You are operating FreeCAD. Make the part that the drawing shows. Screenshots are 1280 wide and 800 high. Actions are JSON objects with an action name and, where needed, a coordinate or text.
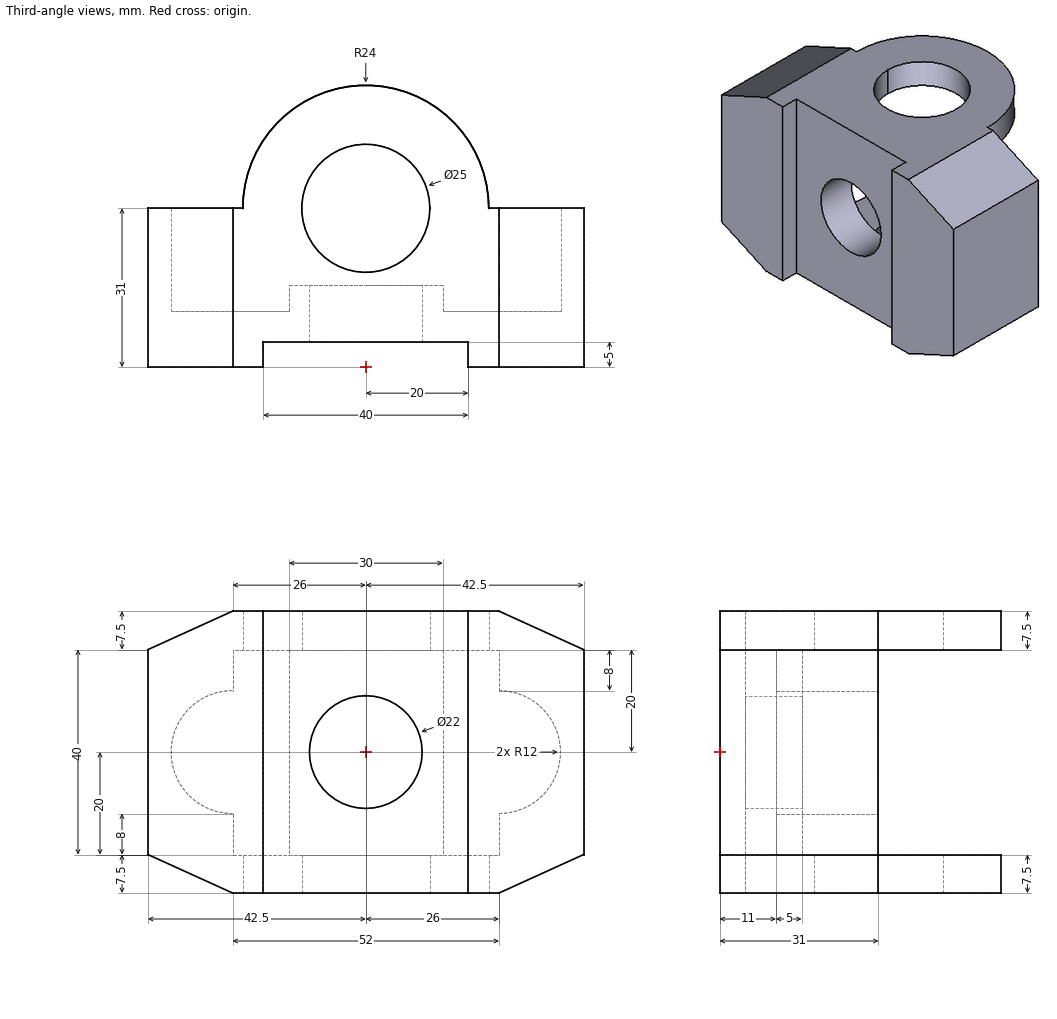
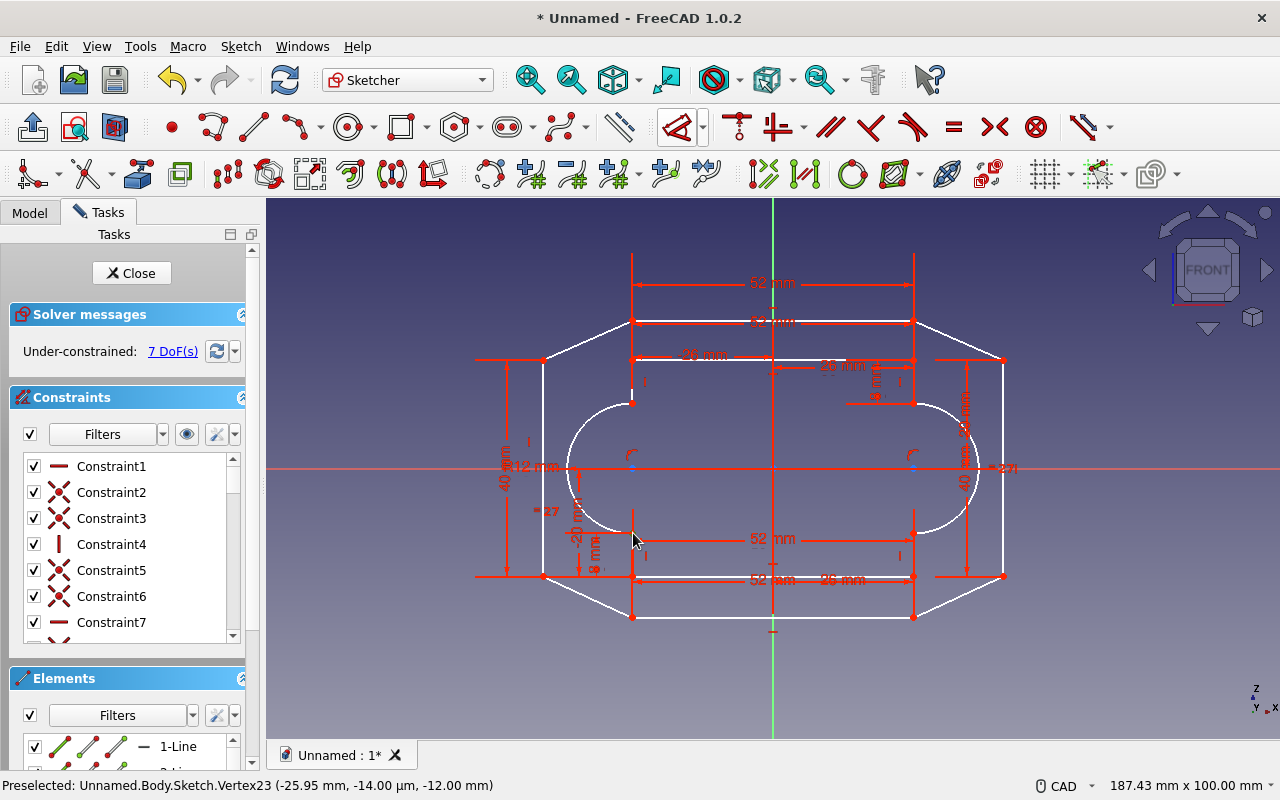
{"action": "key", "text": "l"}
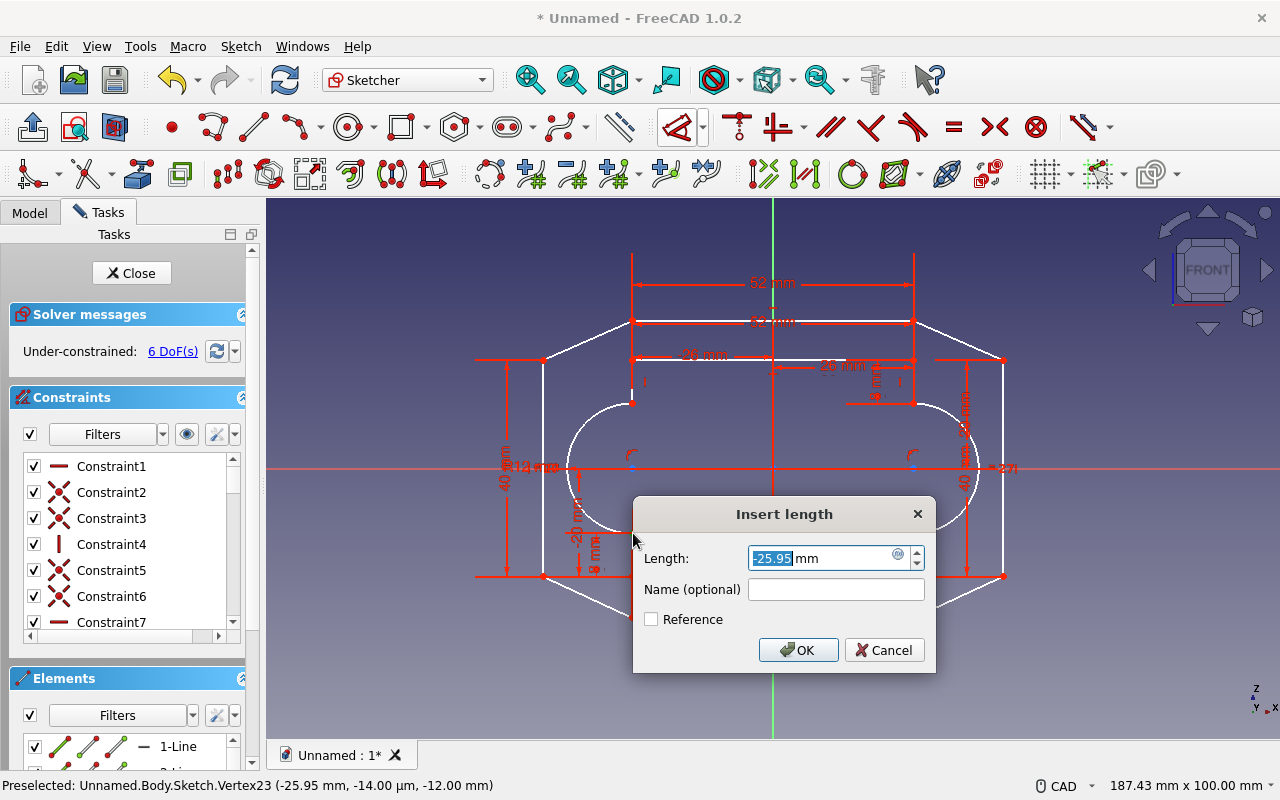
{"action": "type", "text": "-26"}
{"action": "key", "text": "Return"}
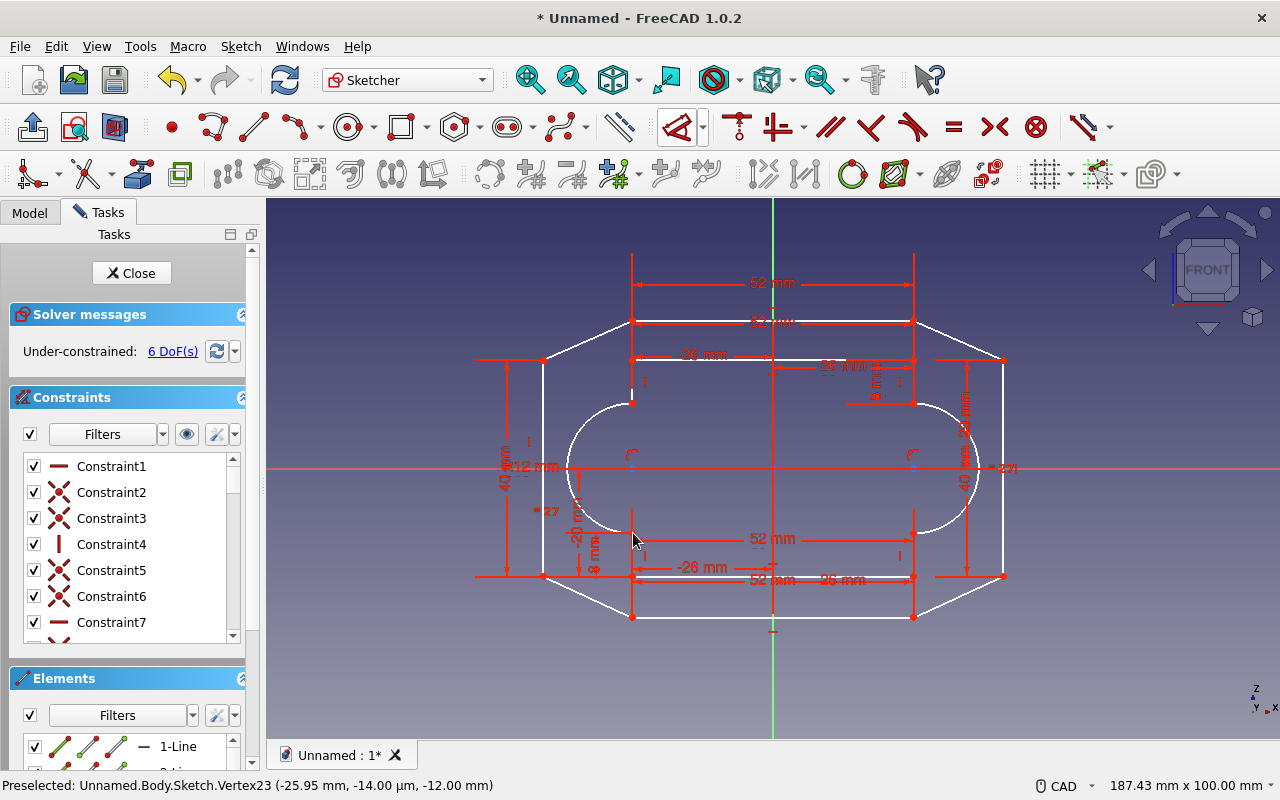
{"action": "left_click", "coordinate": [632, 468]}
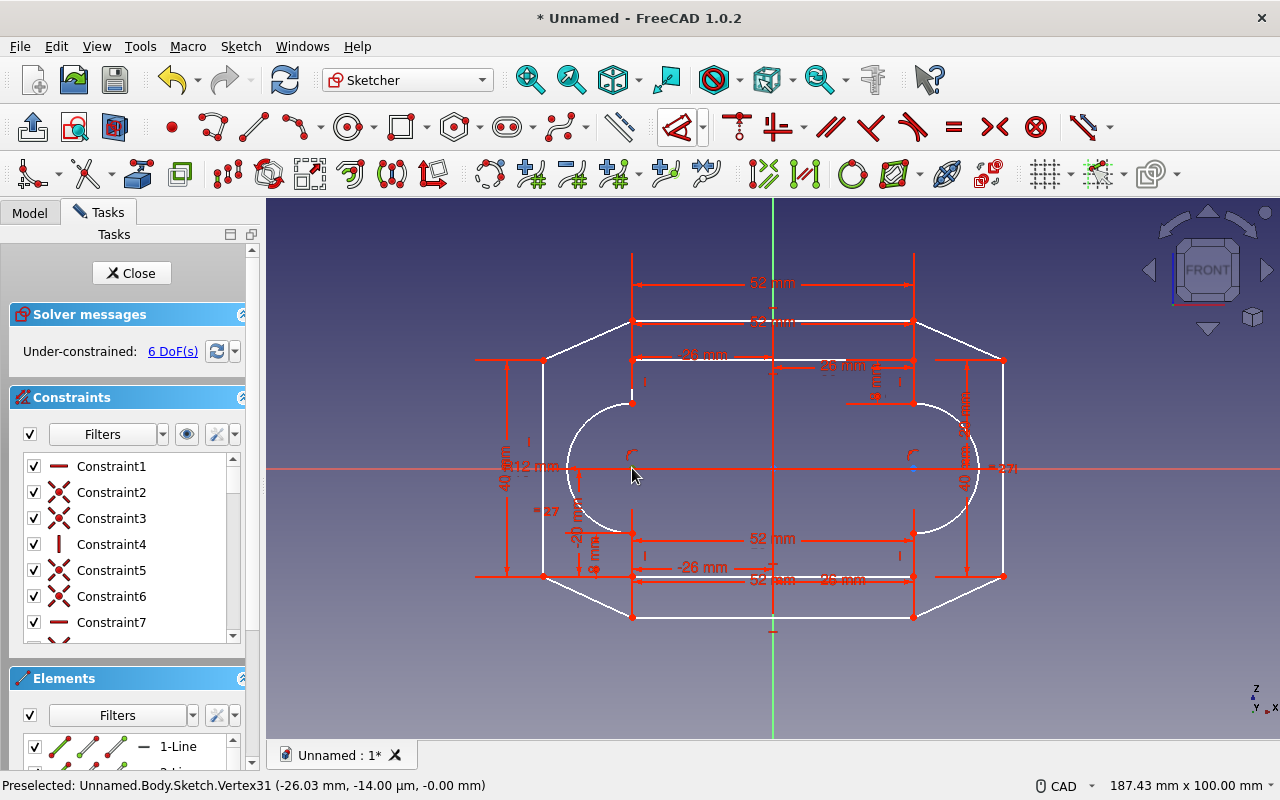
{"action": "left_click", "coordinate": [702, 128]}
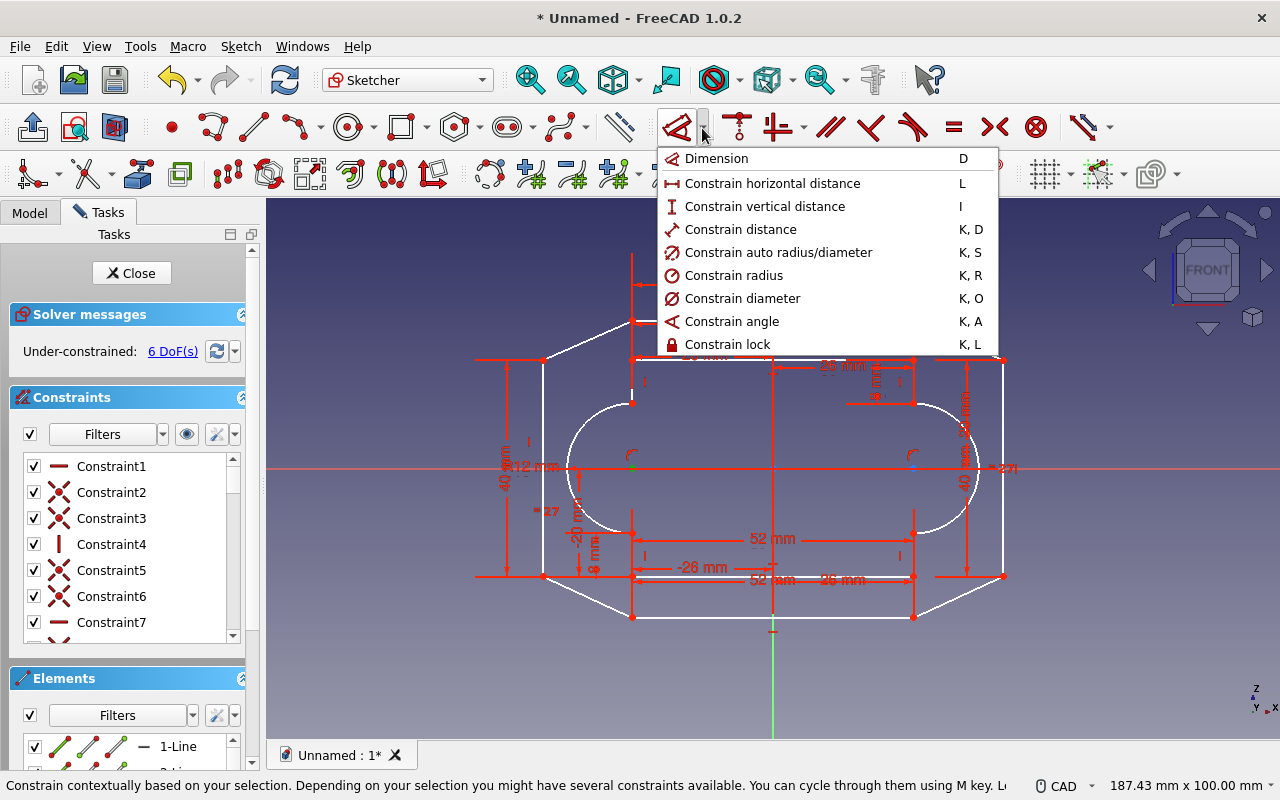
{"action": "left_click", "coordinate": [828, 184]}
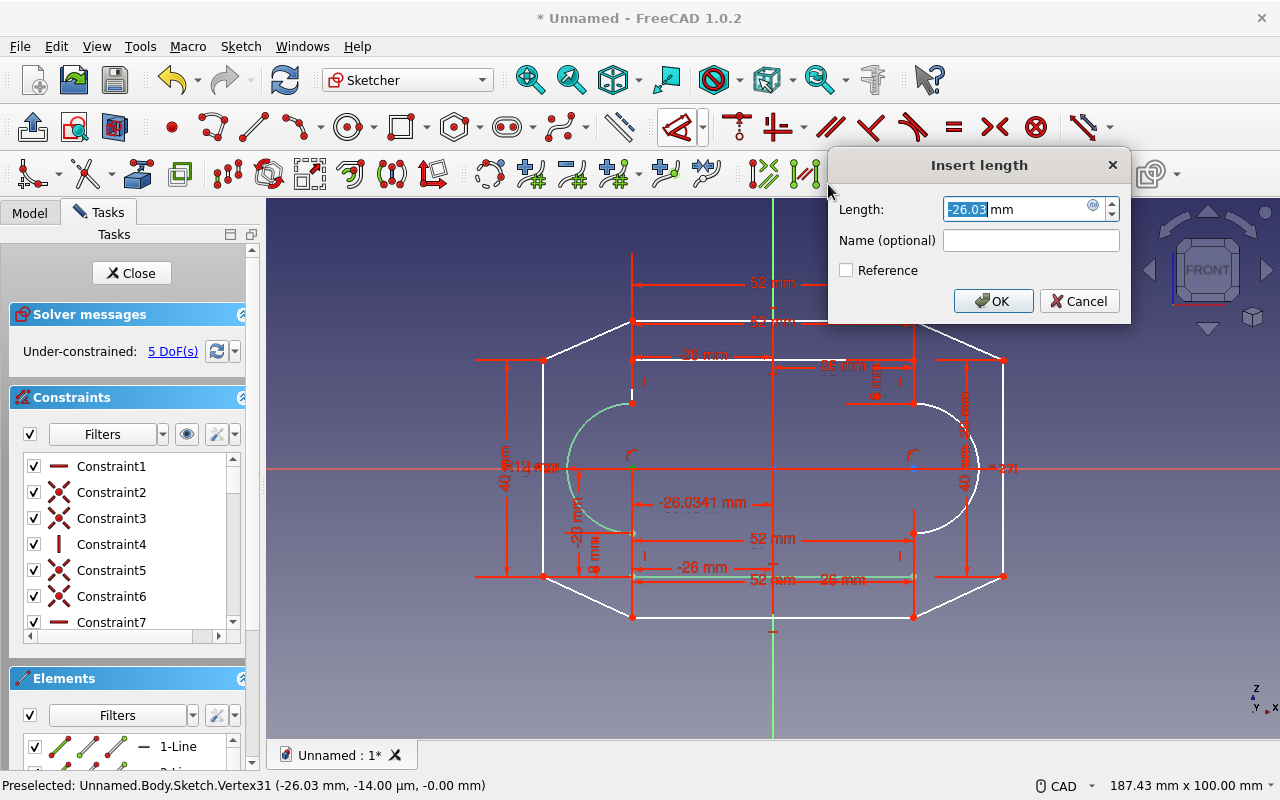
{"action": "type", "text": "-26"}
{"action": "key", "text": "Return"}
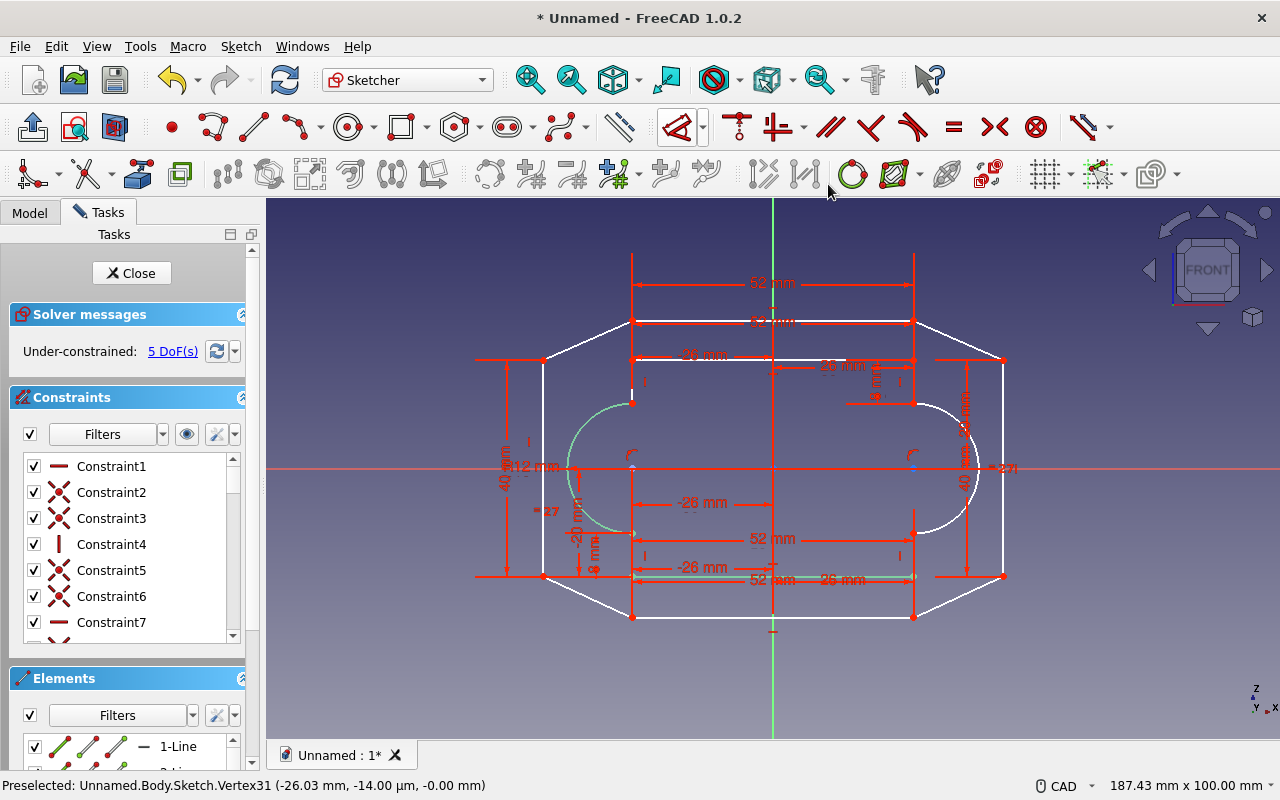
{"action": "left_click", "coordinate": [914, 468]}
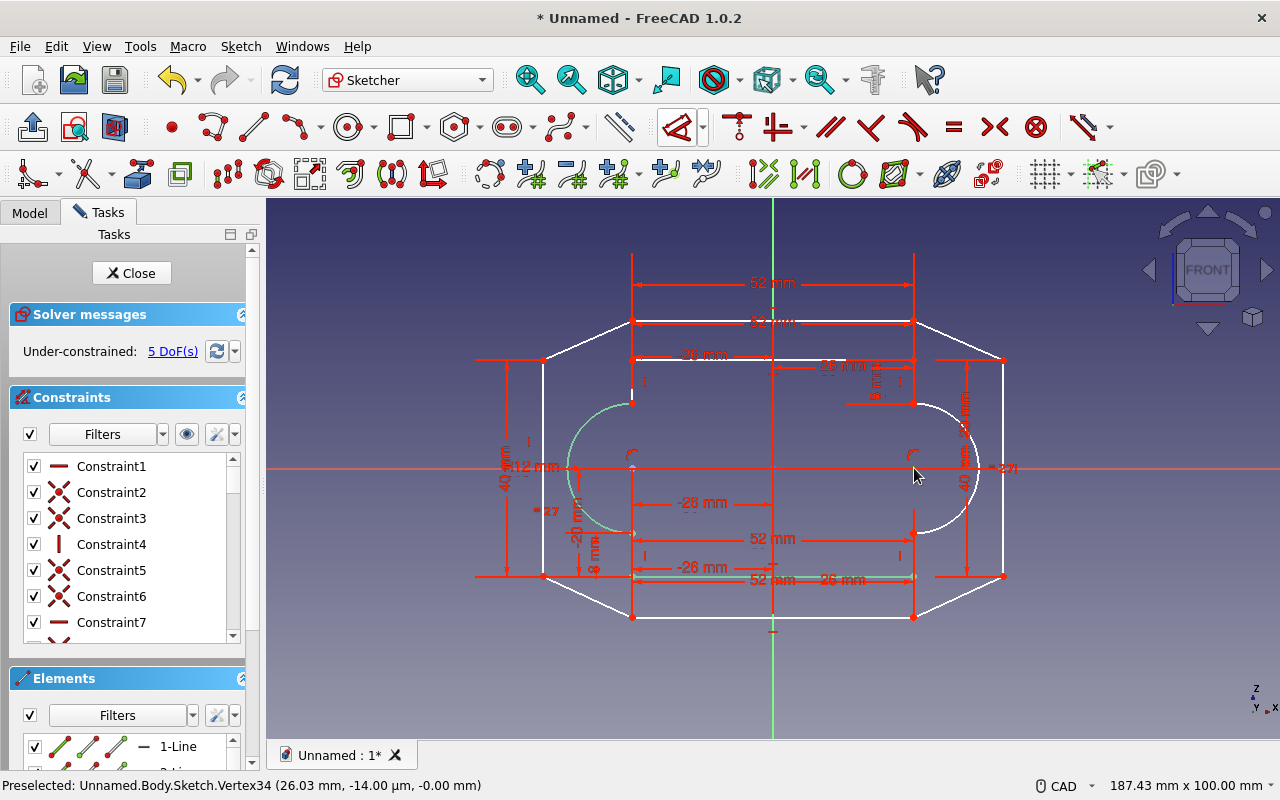
{"action": "key", "text": "l"}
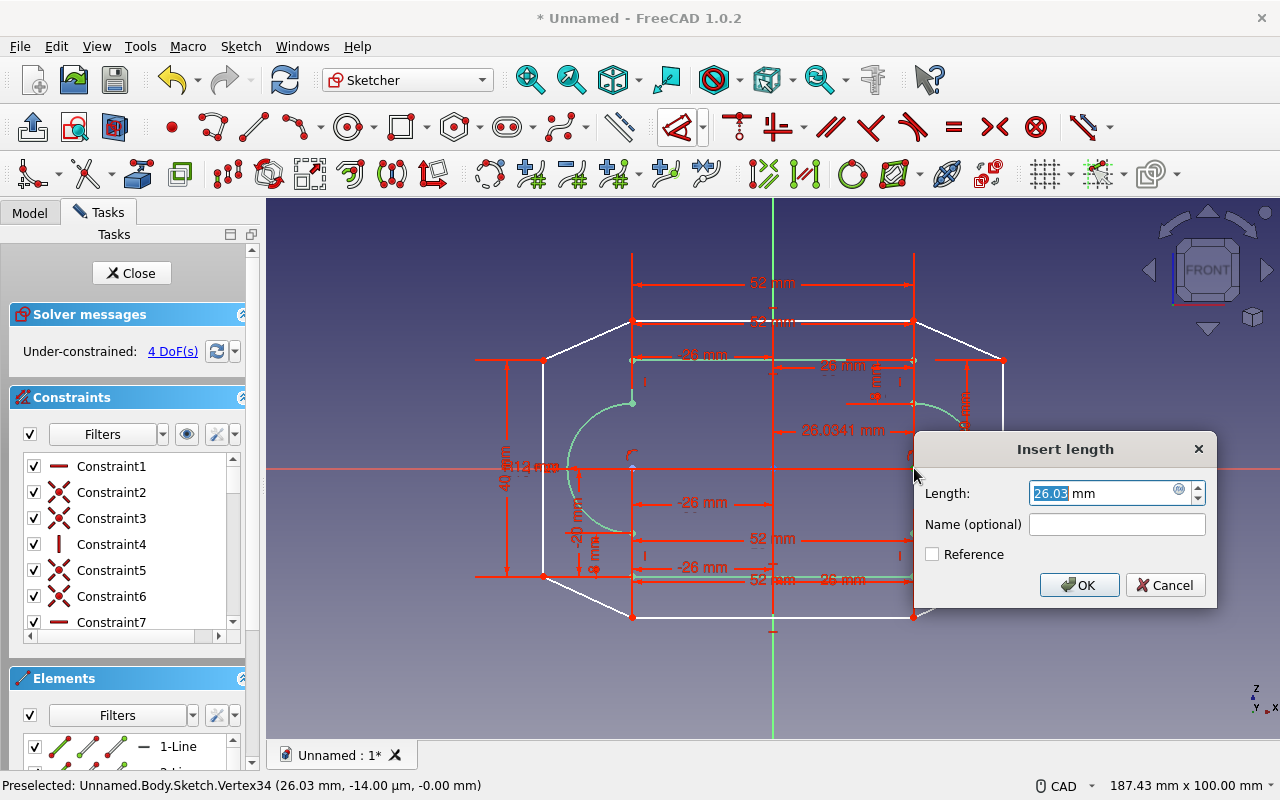
{"action": "type", "text": "26"}
{"action": "key", "text": "Return"}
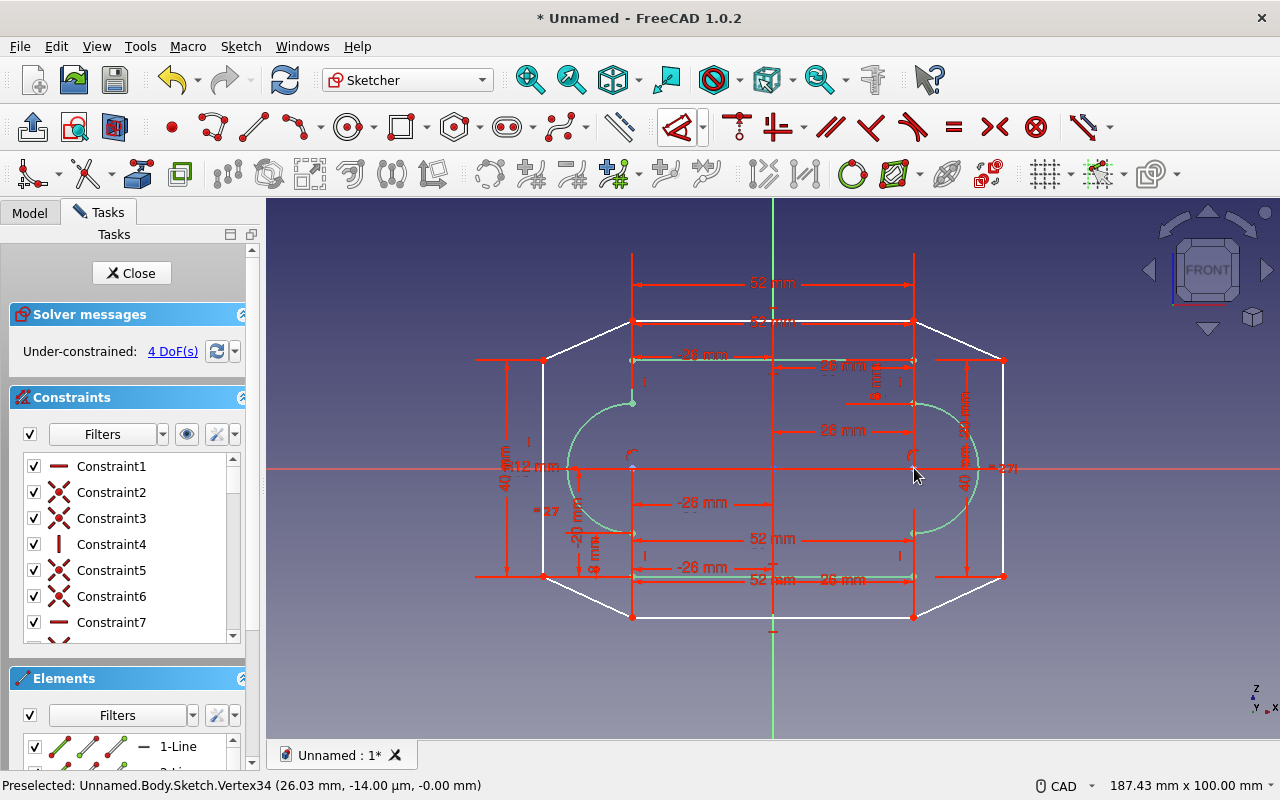
{"action": "left_click", "coordinate": [606, 606]}